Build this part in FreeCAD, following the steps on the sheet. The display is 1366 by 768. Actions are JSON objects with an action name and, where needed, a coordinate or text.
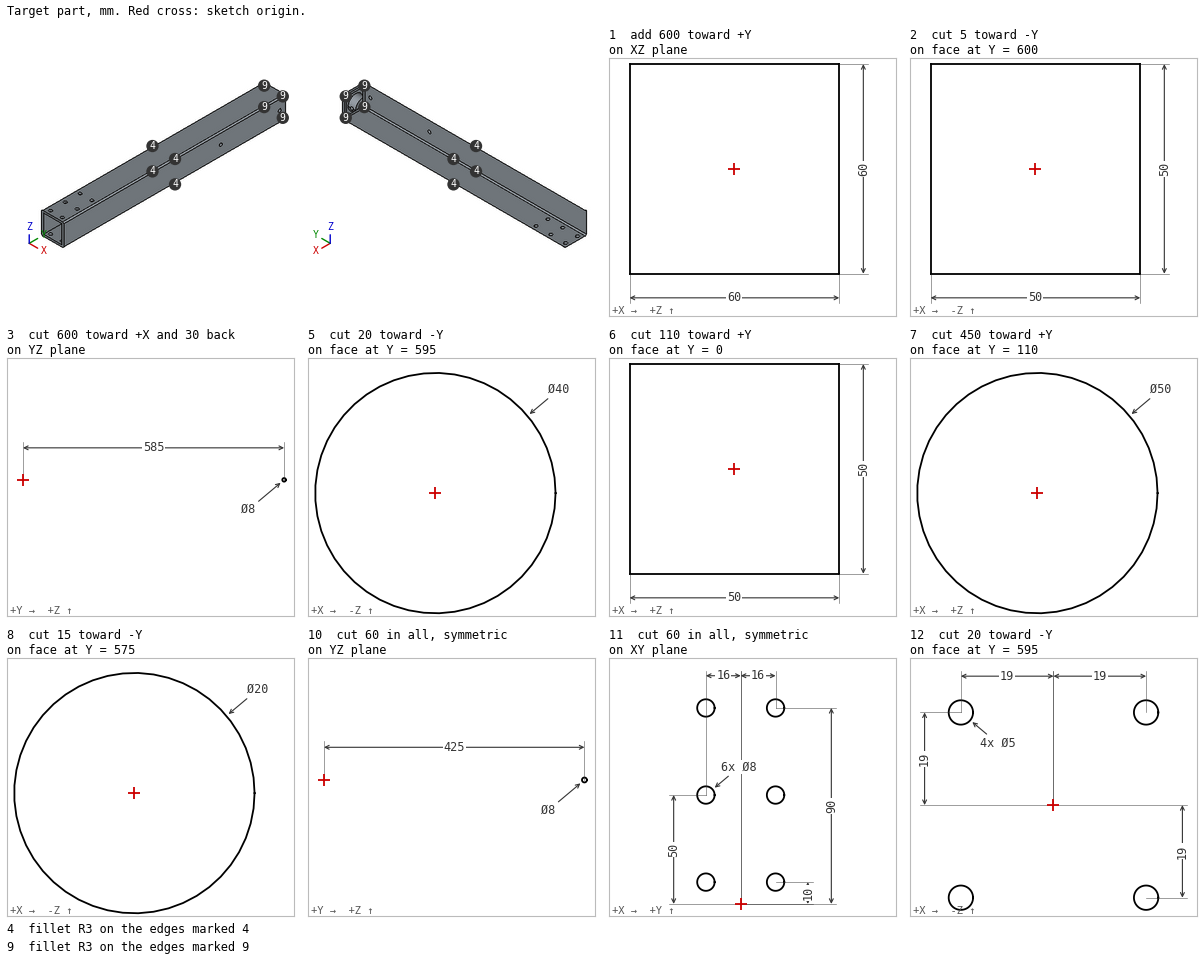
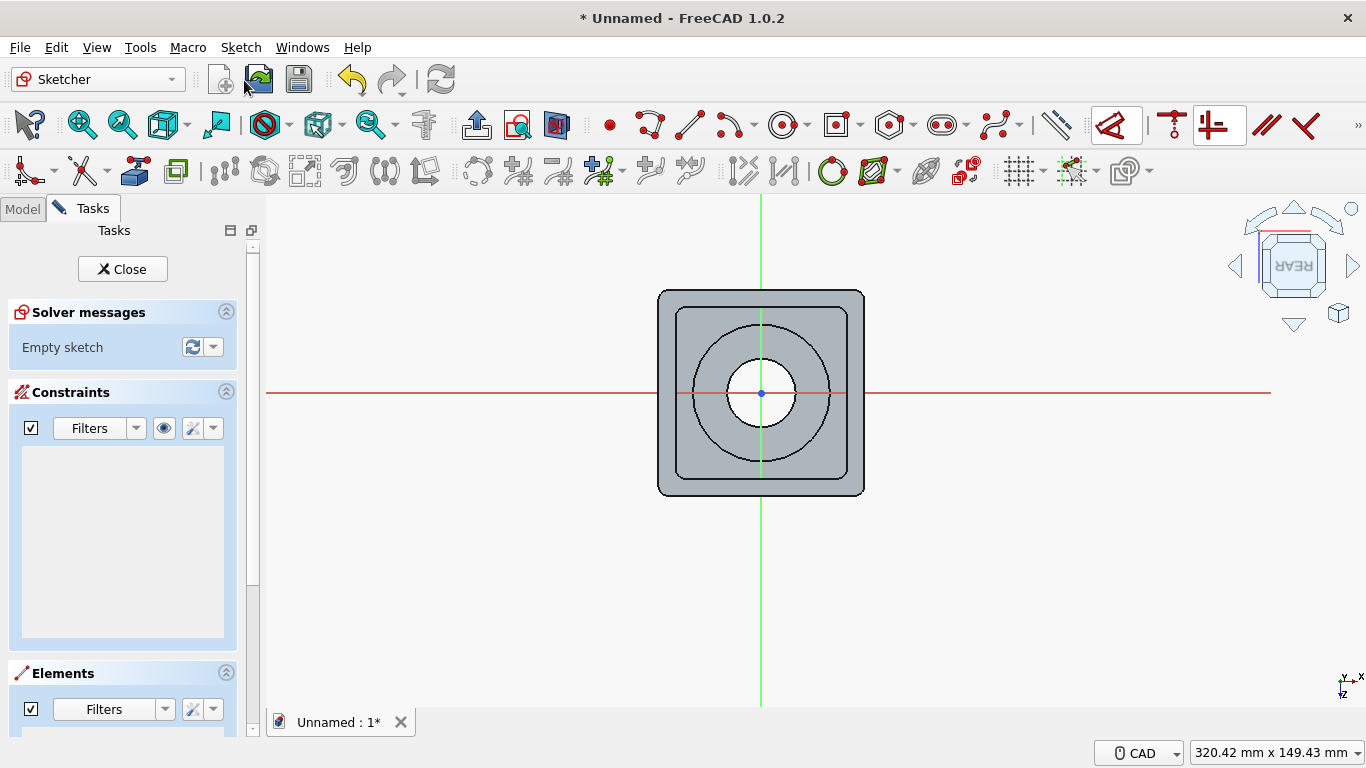
{"action": "left_click", "coordinate": [558, 126]}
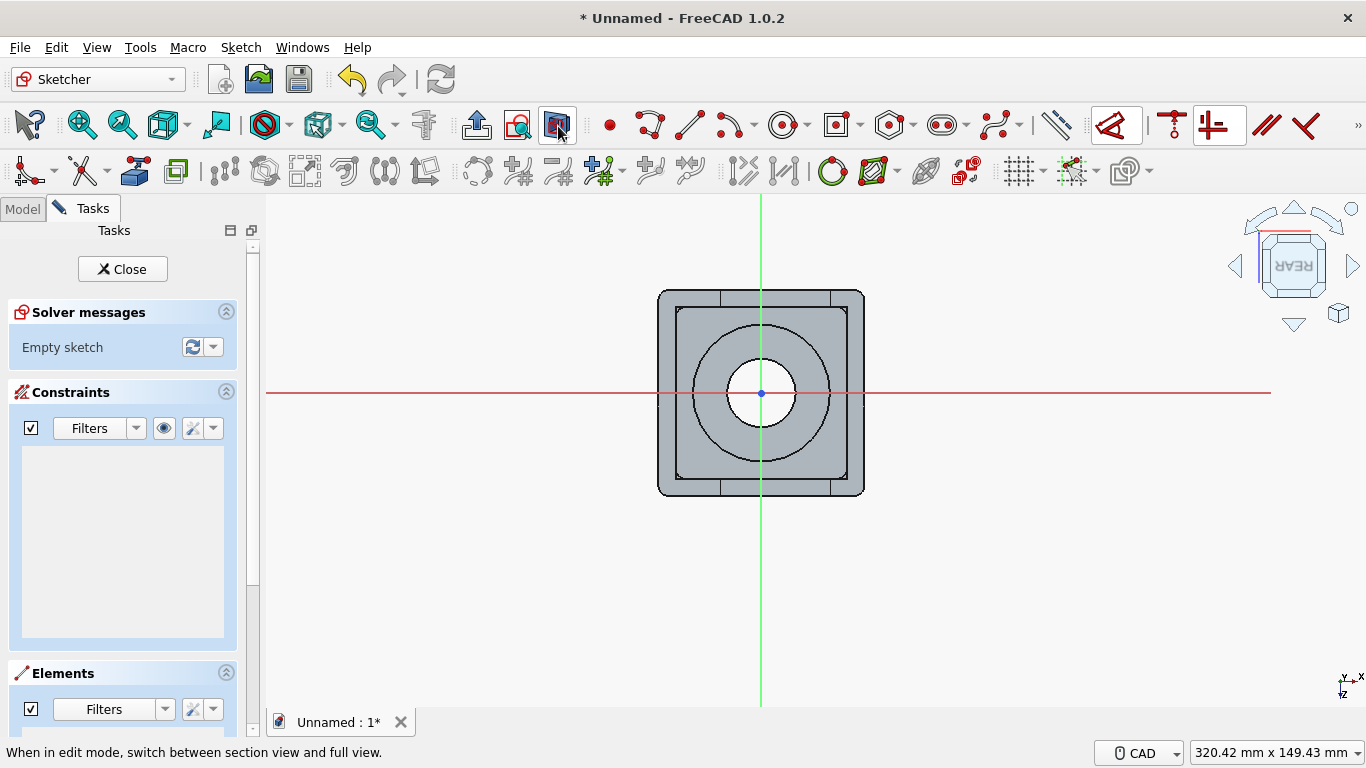
{"action": "scroll", "coordinate": [773, 346], "scroll_direction": "up", "scroll_amount": 4}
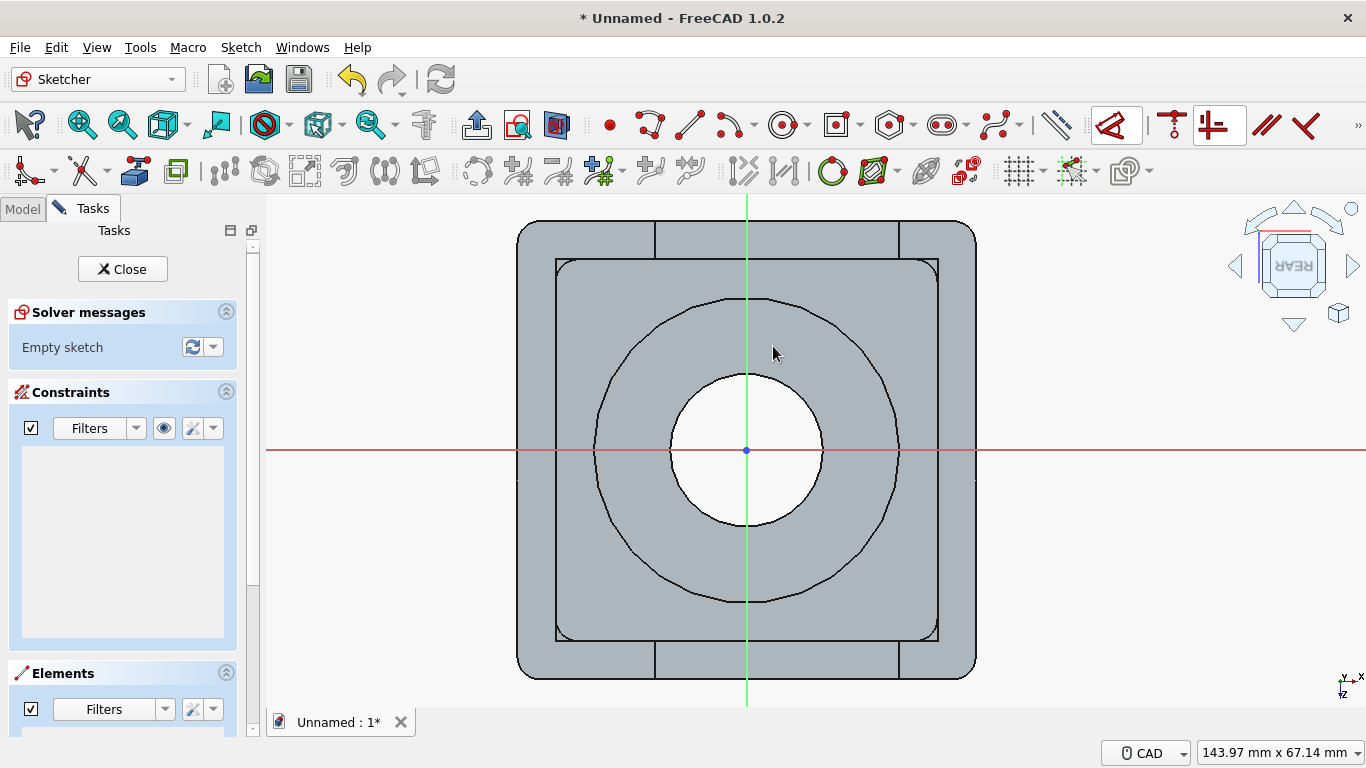
{"action": "left_click", "coordinate": [784, 126]}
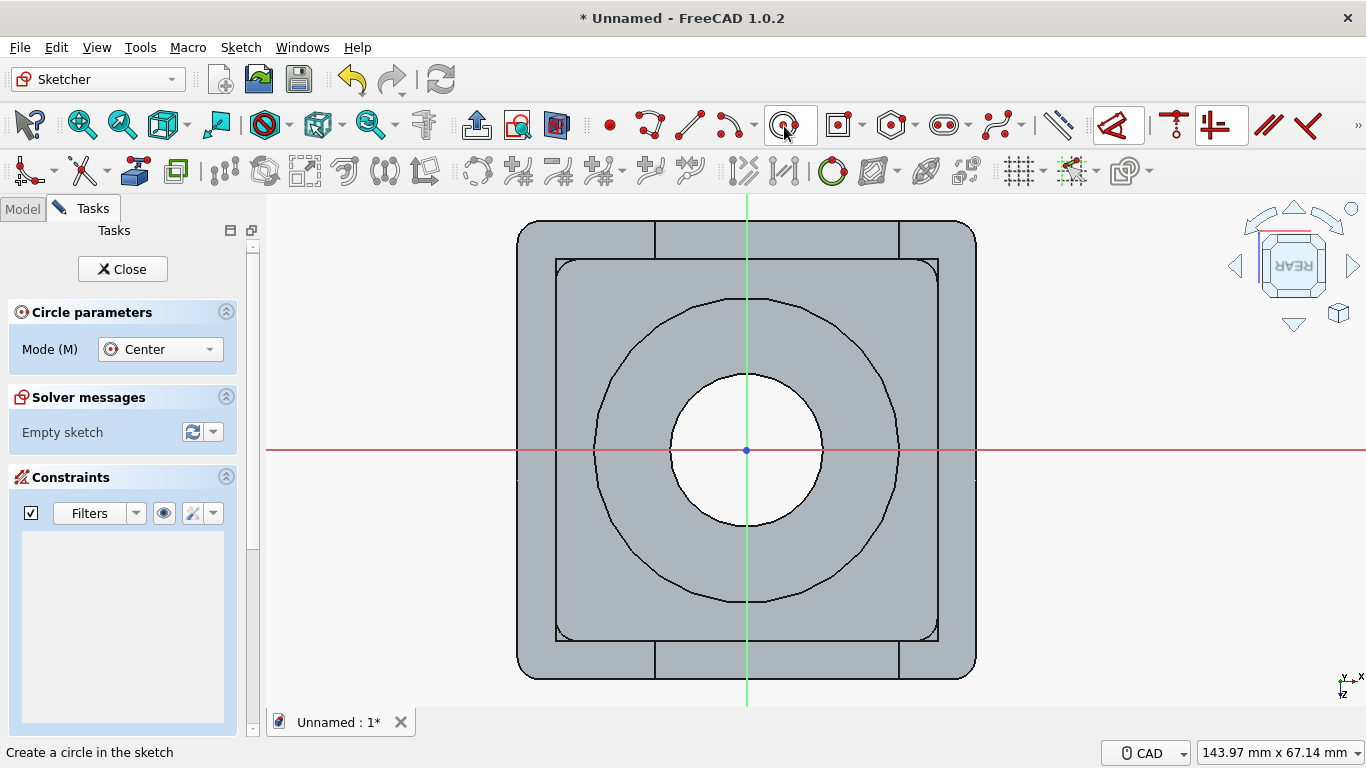
{"action": "left_click", "coordinate": [601, 305]}
{"action": "mouse_move", "coordinate": [615, 292]}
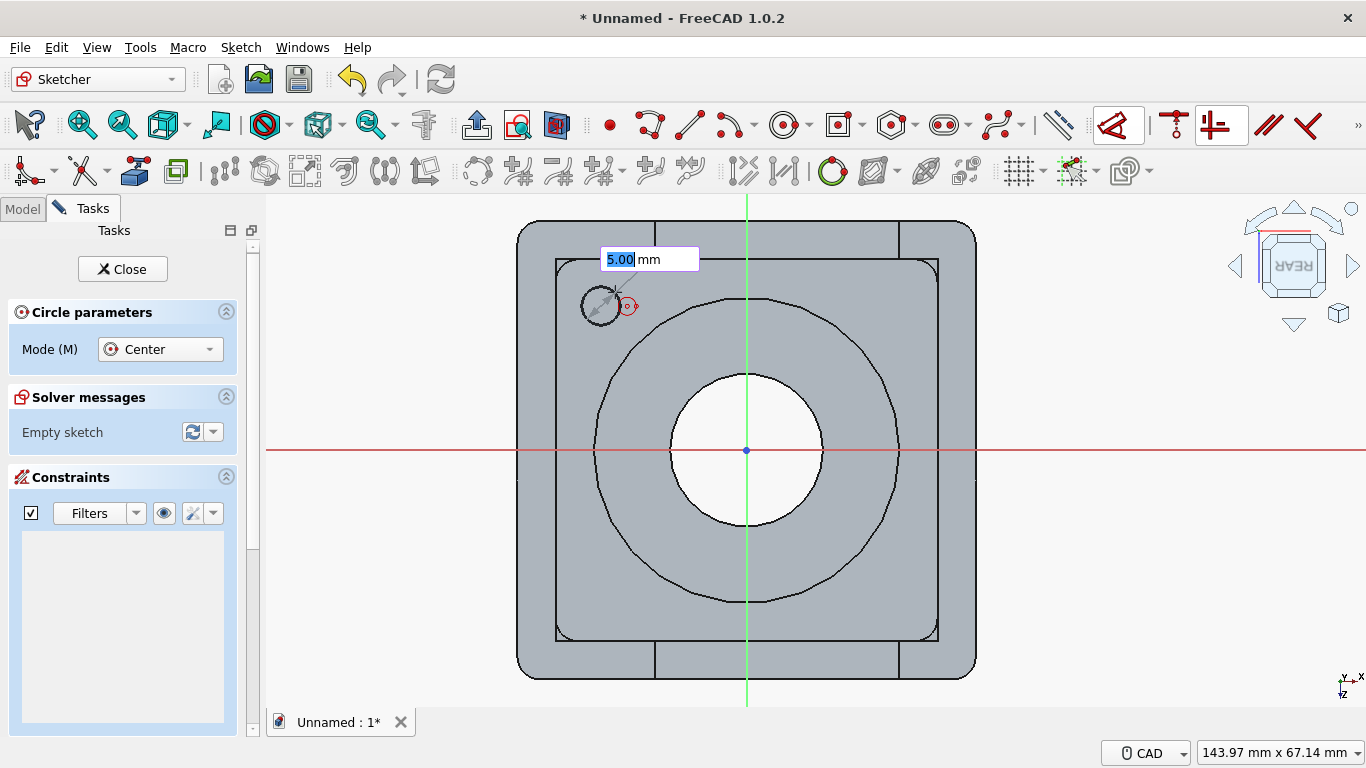
{"action": "type", "text": "5"}
{"action": "key", "text": "Return"}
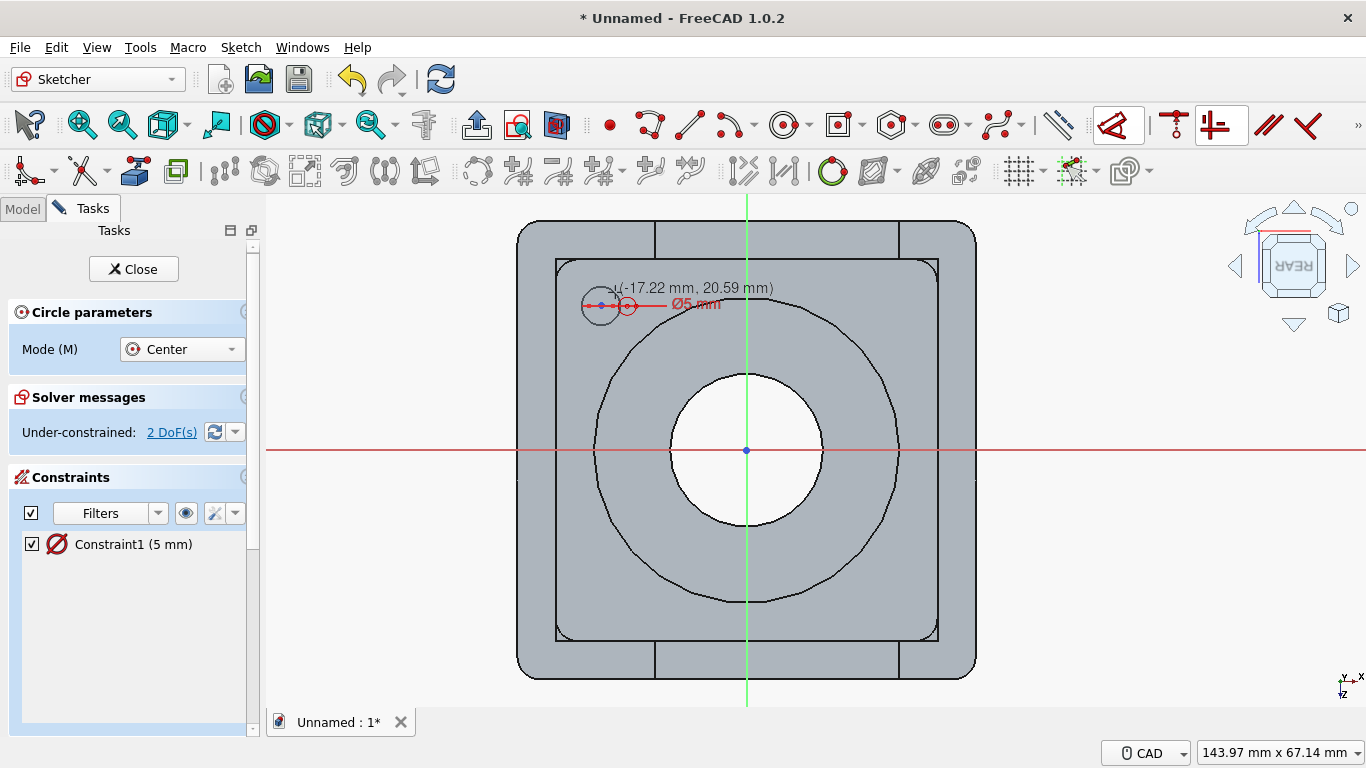
{"action": "left_click", "coordinate": [892, 305]}
{"action": "mouse_move", "coordinate": [905, 292]}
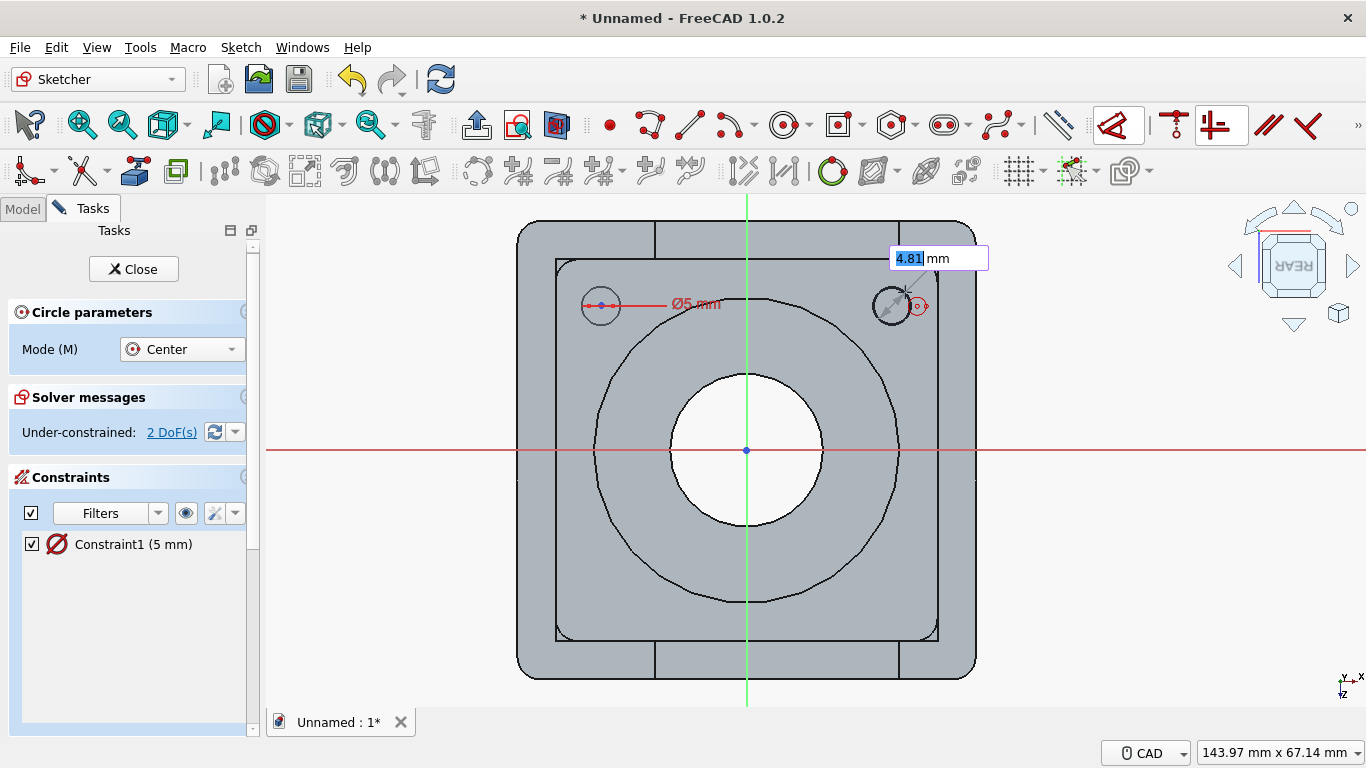
{"action": "type", "text": "5"}
{"action": "key", "text": "Return"}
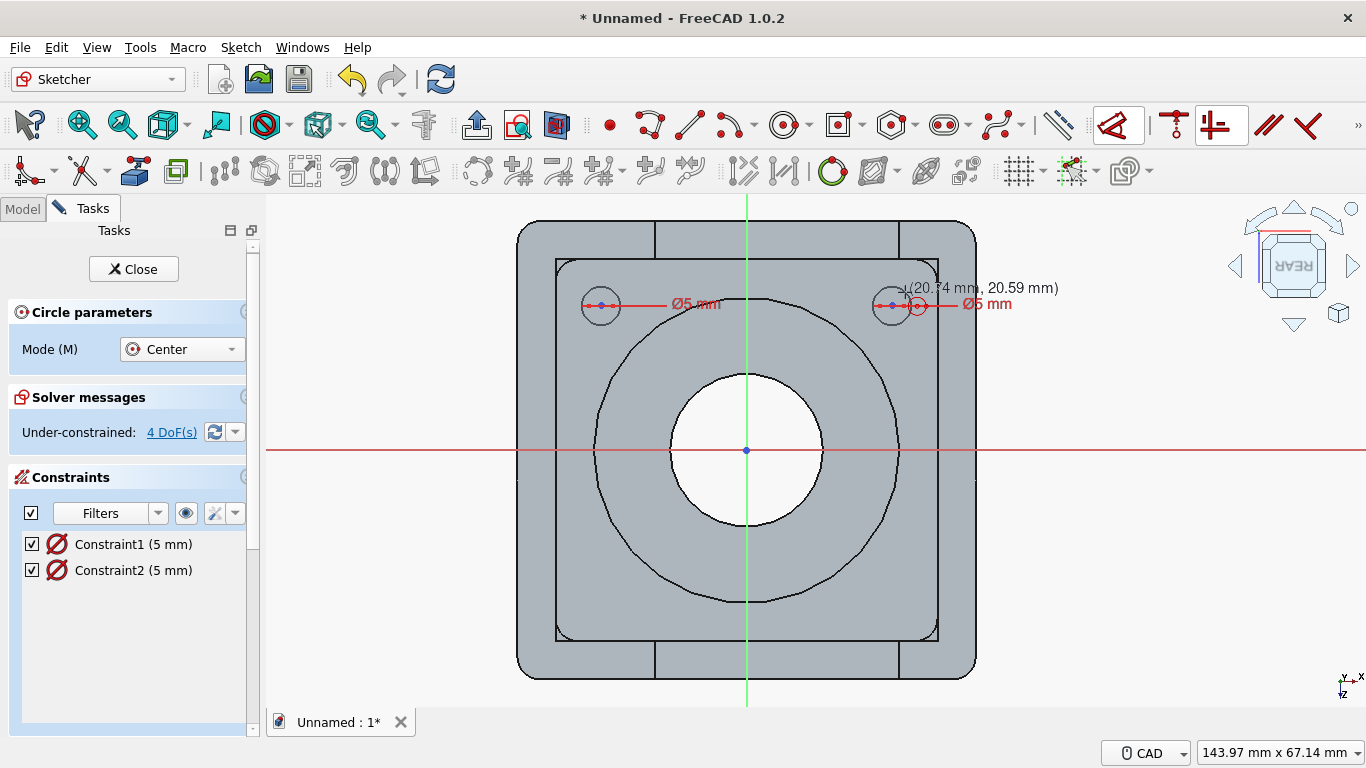
{"action": "left_click", "coordinate": [892, 595]}
{"action": "mouse_move", "coordinate": [905, 582]}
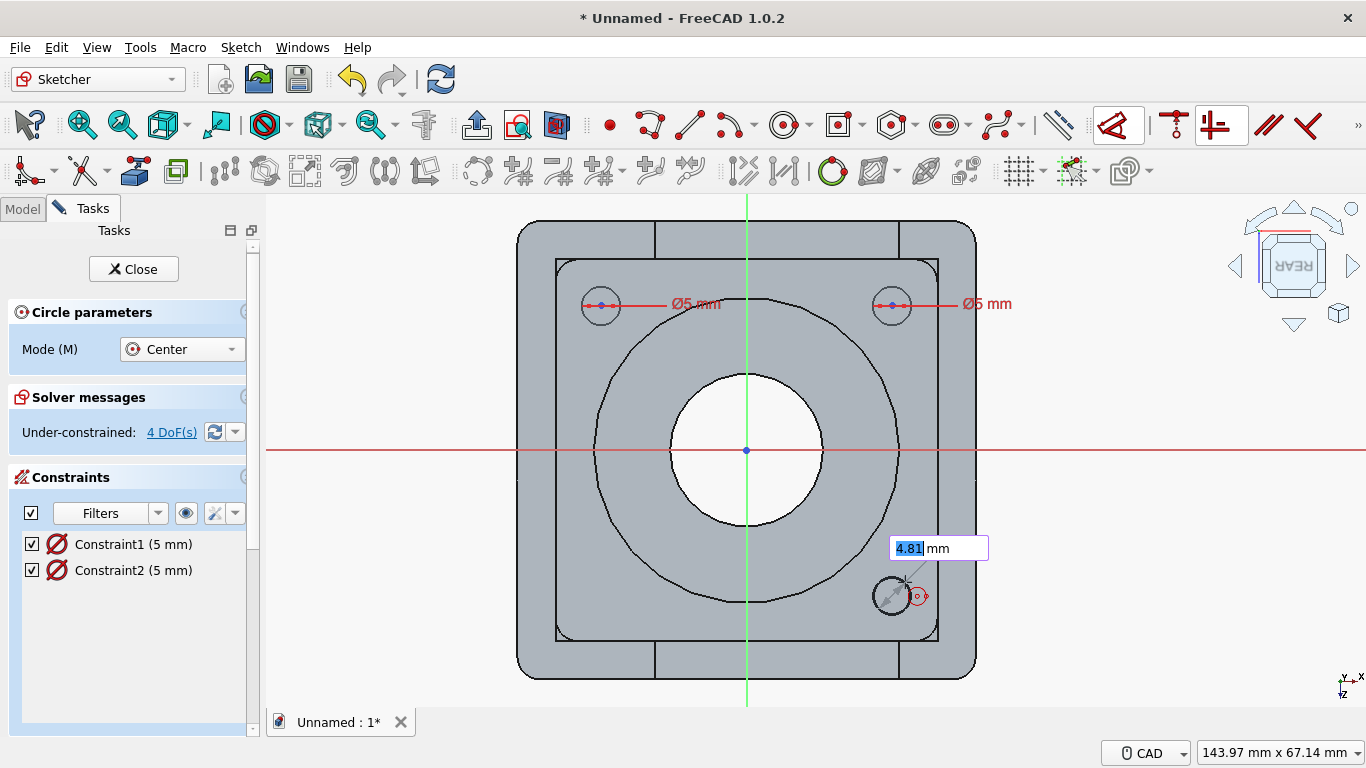
{"action": "type", "text": "5"}
{"action": "key", "text": "Return"}